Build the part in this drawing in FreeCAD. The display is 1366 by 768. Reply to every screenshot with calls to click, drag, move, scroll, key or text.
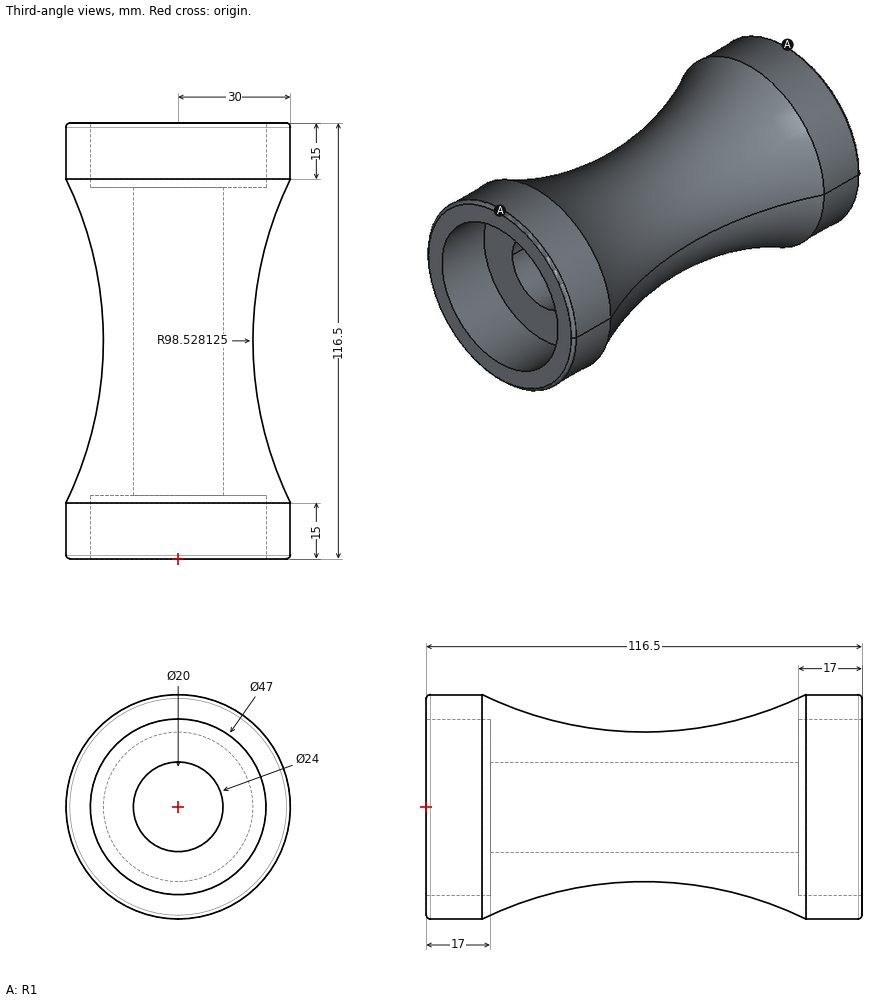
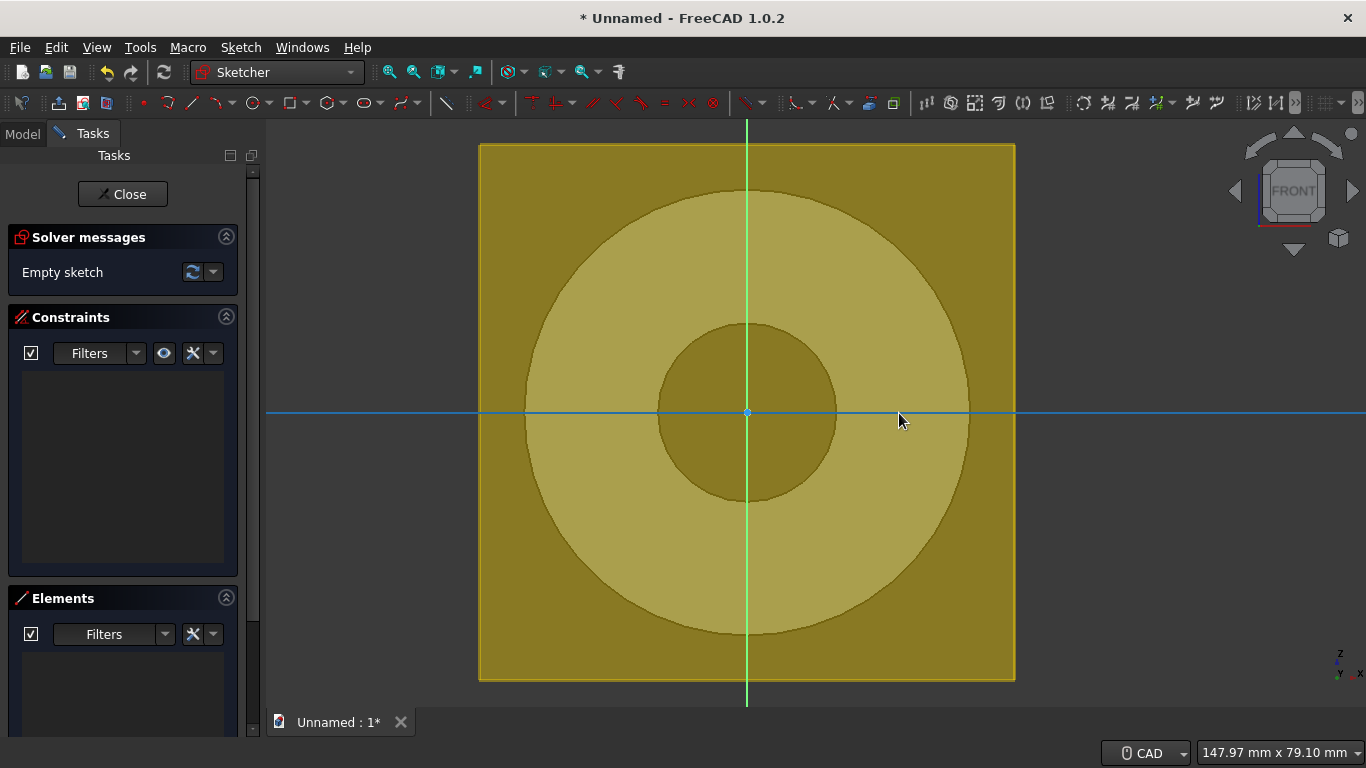
click(254, 104)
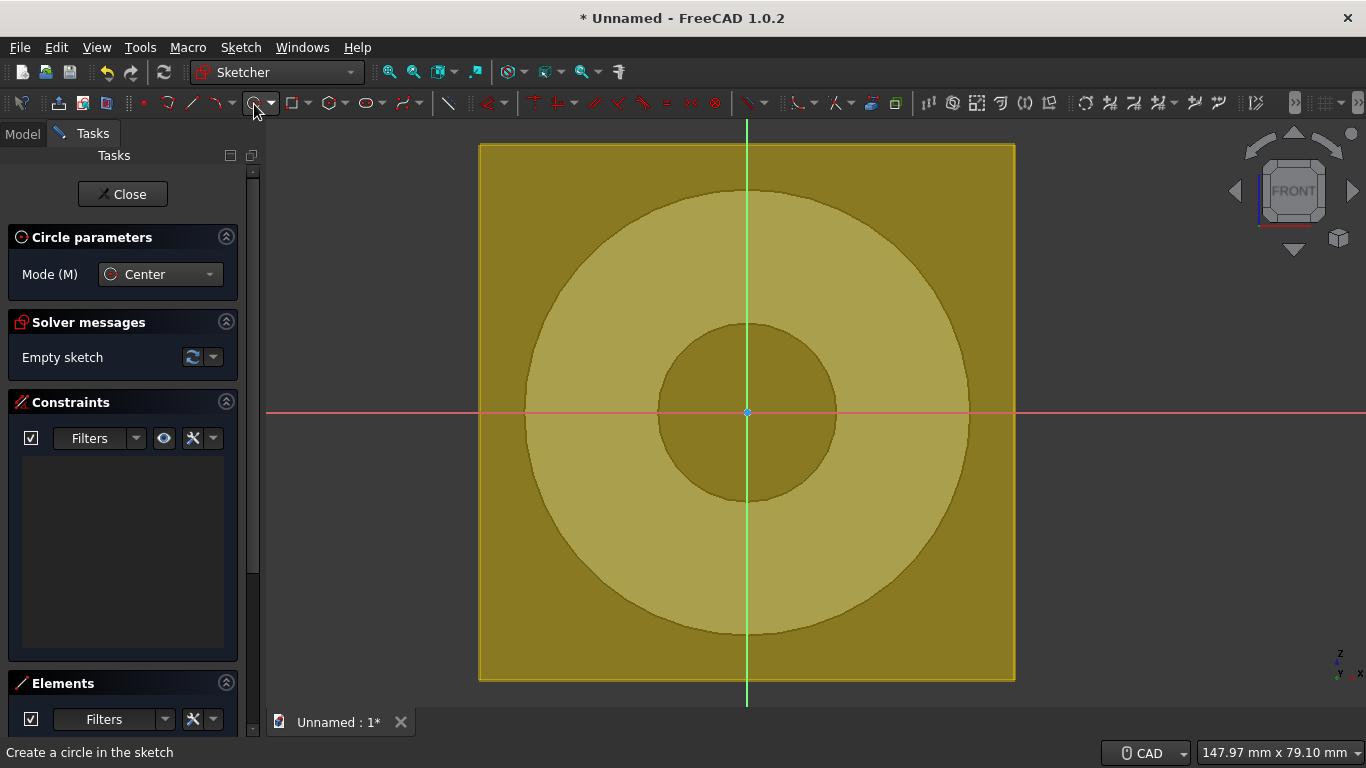
click(747, 413)
click(871, 289)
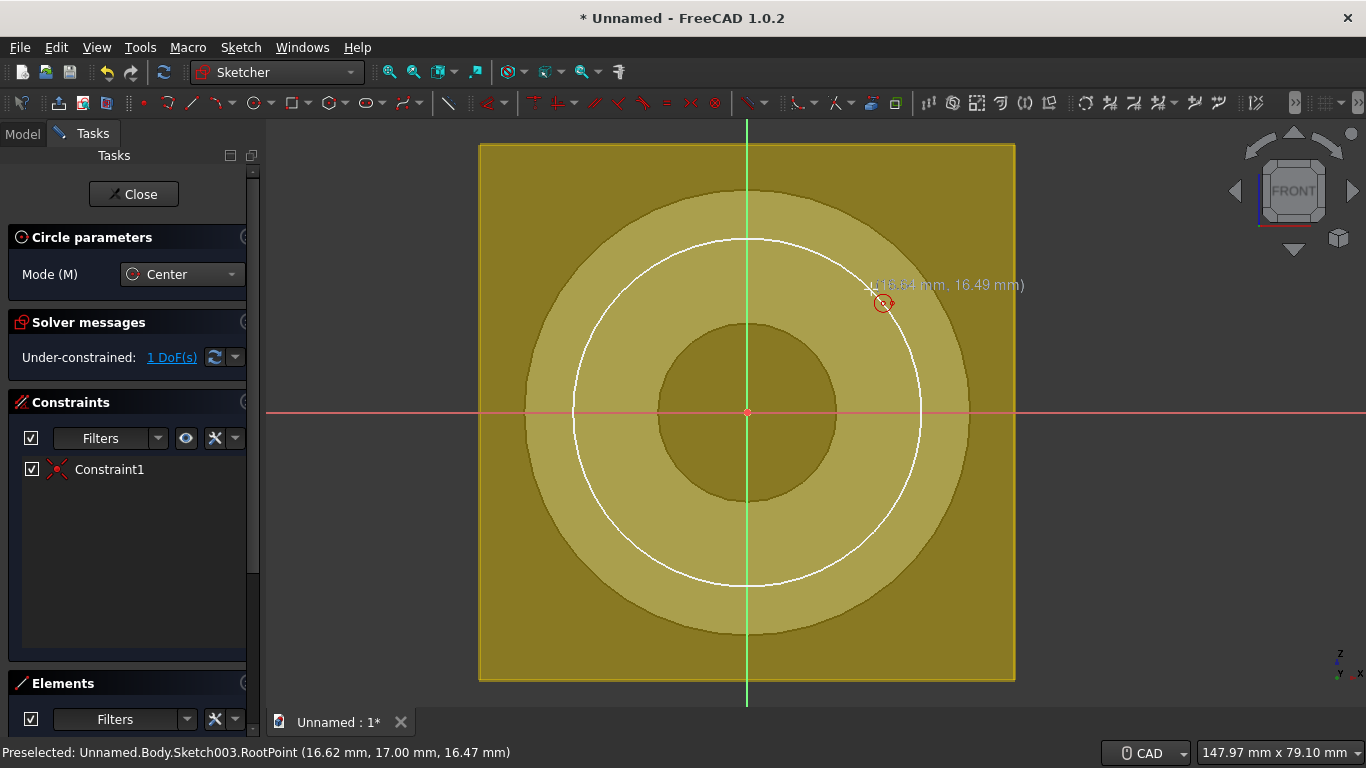
click(747, 413)
click(800, 360)
key(Escape)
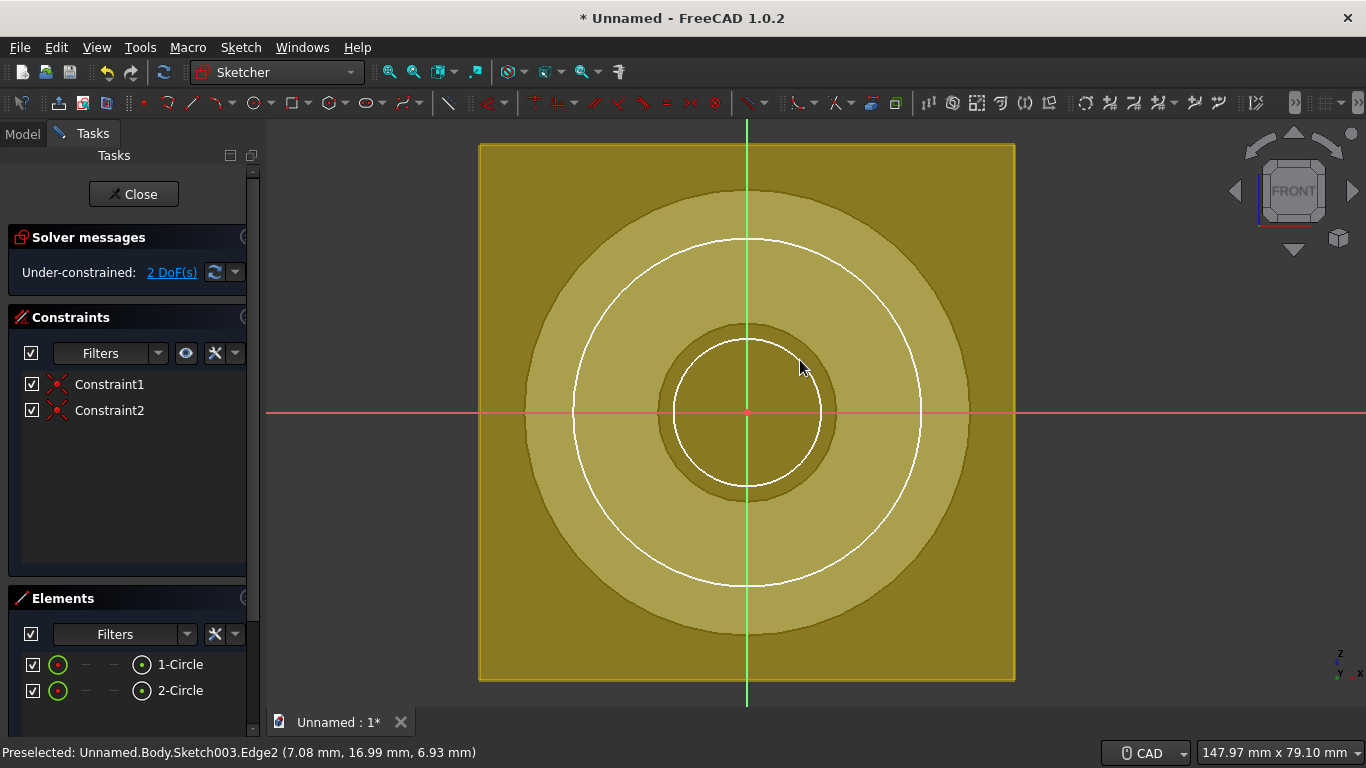
click(488, 104)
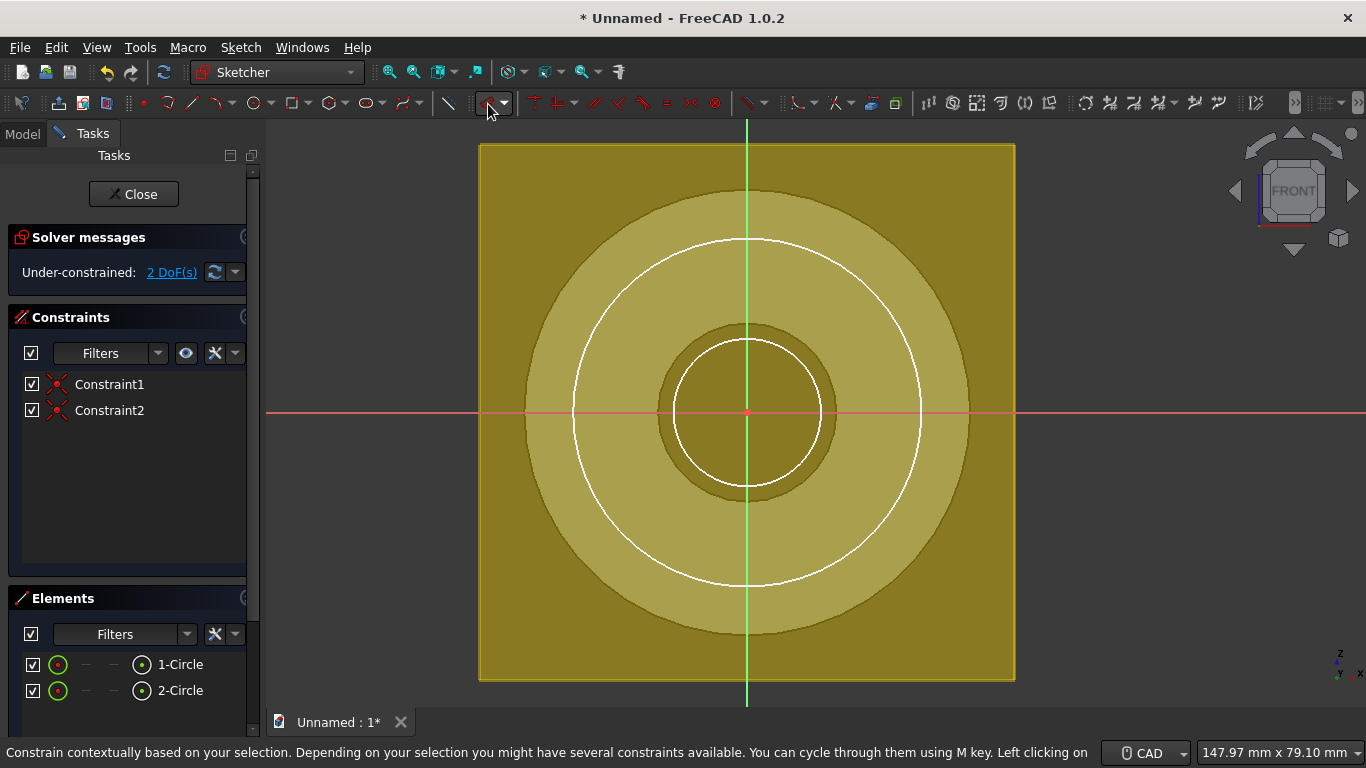
click(870, 289)
click(893, 266)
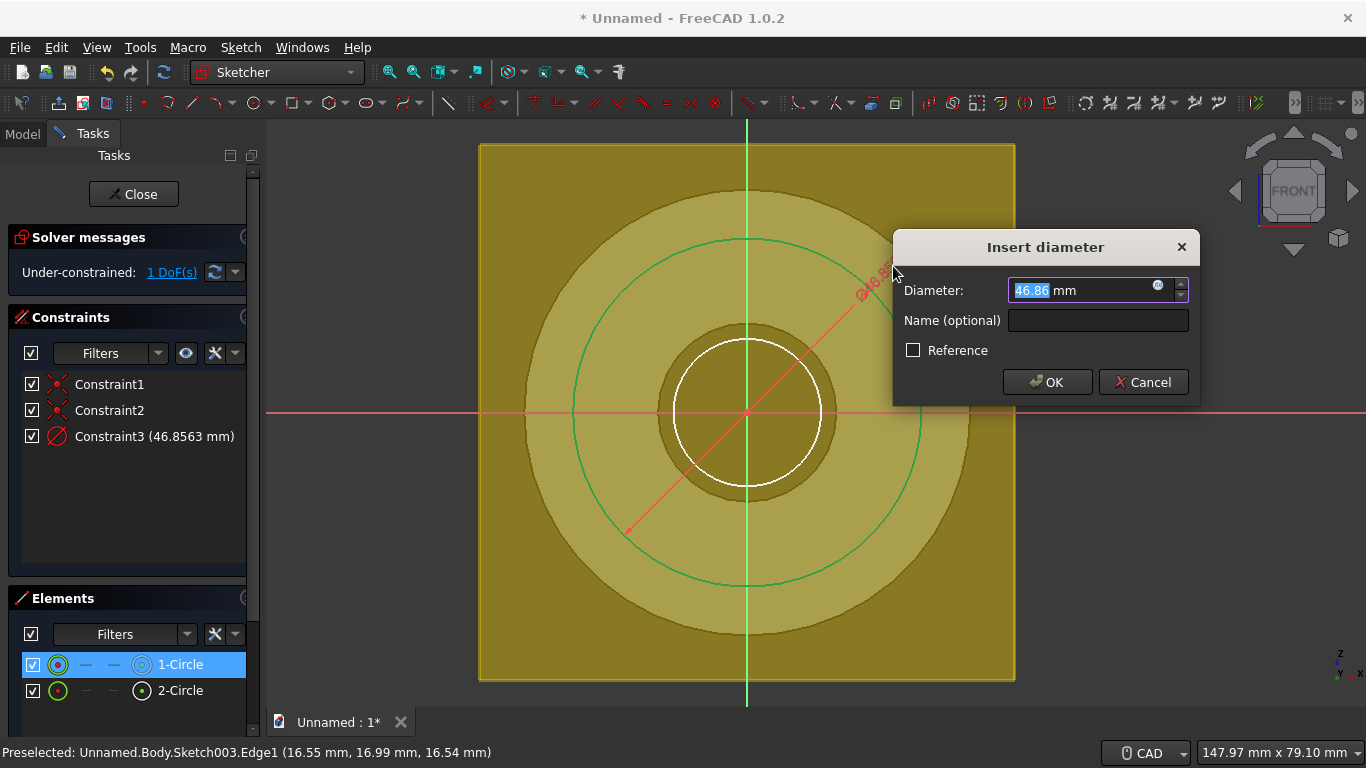
text(47)
key(Return)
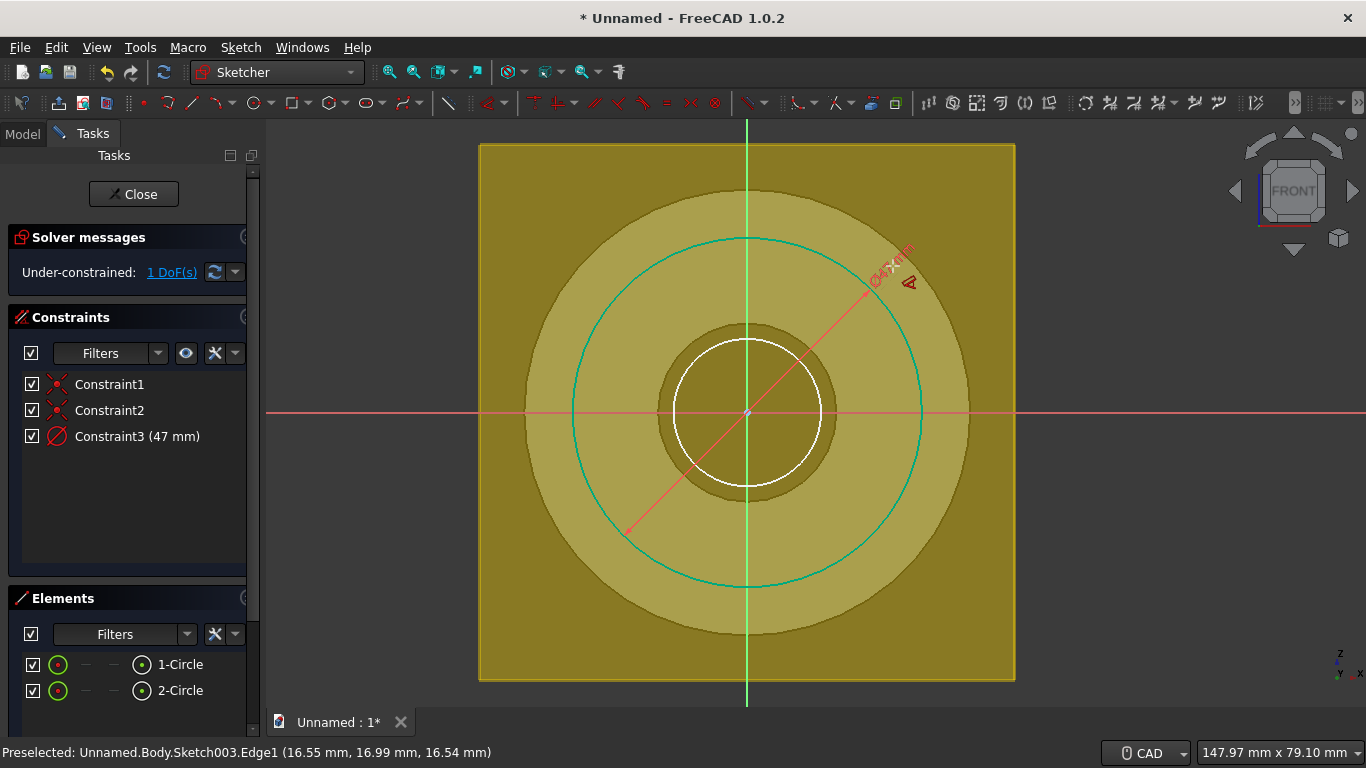
click(799, 360)
click(821, 337)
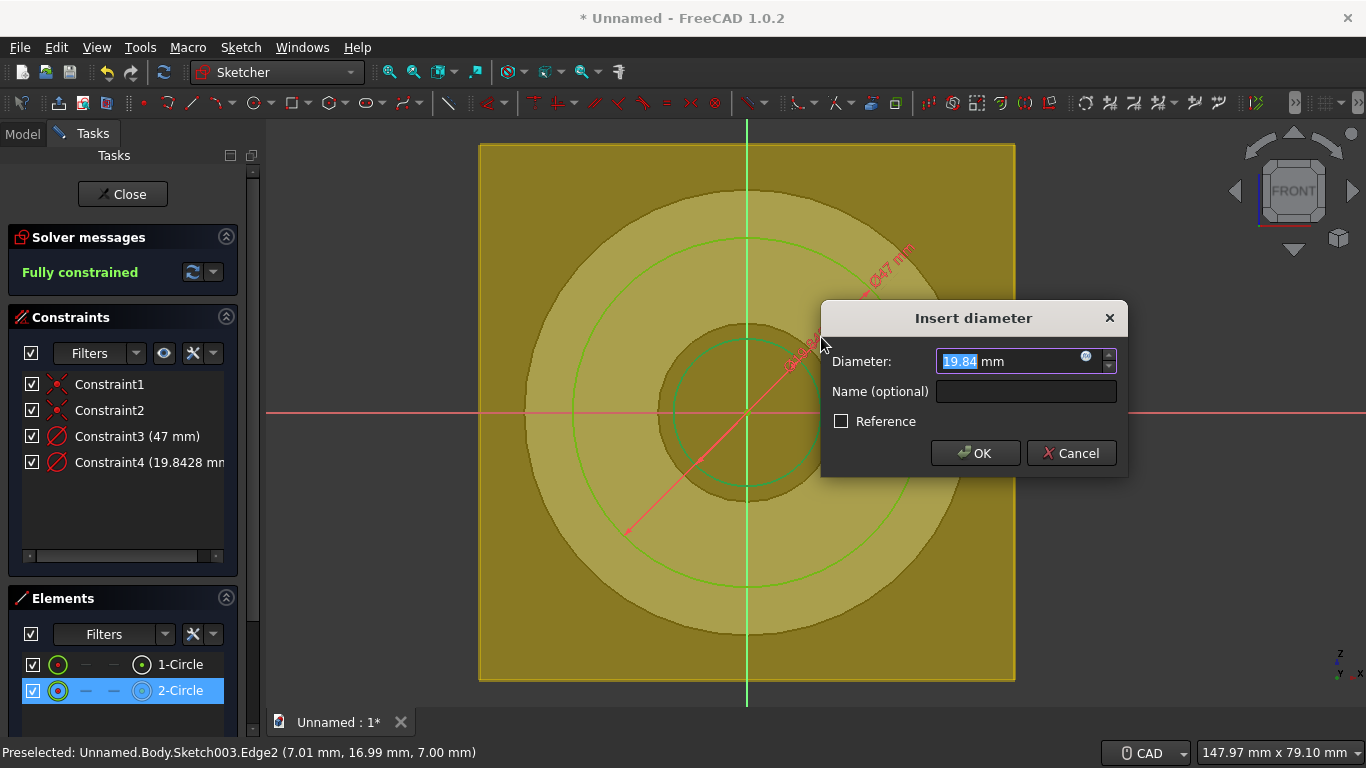
text(20)
key(Return)
key(Escape)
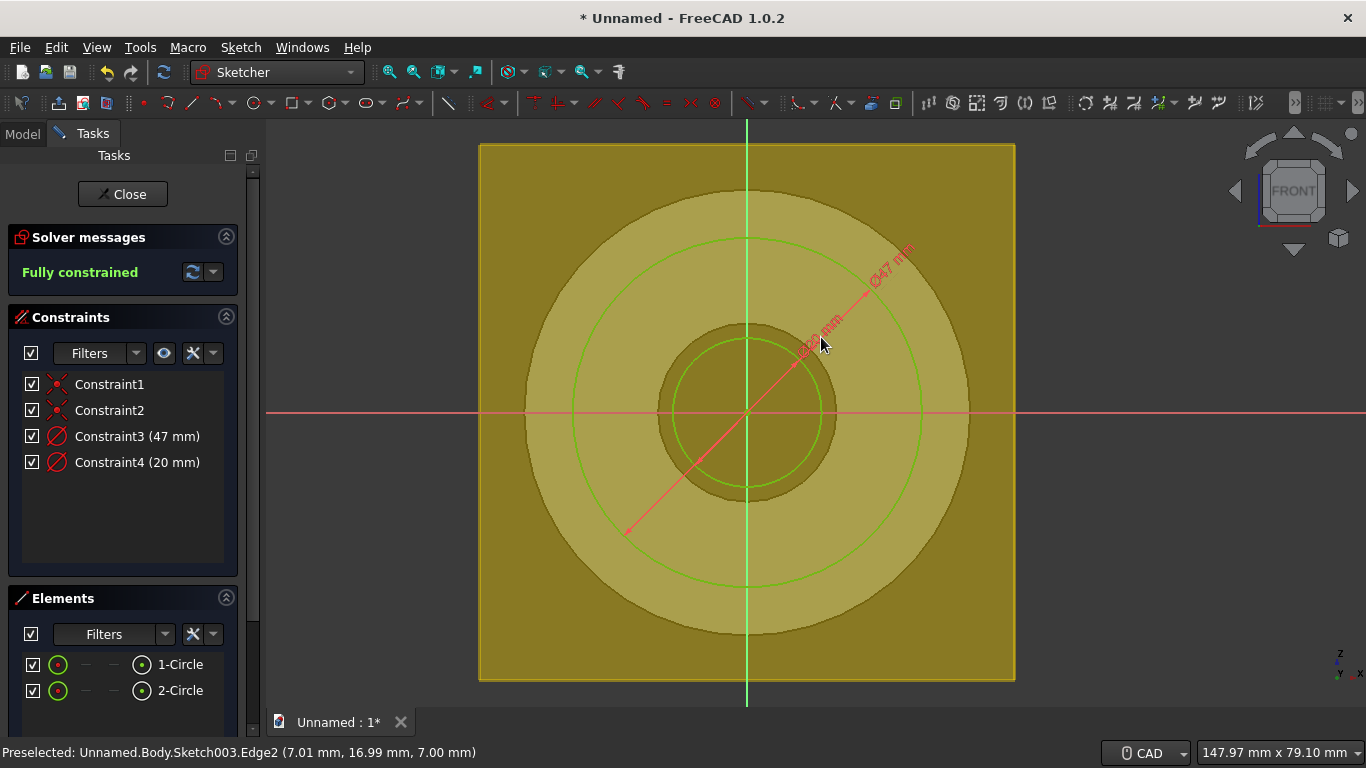
click(123, 194)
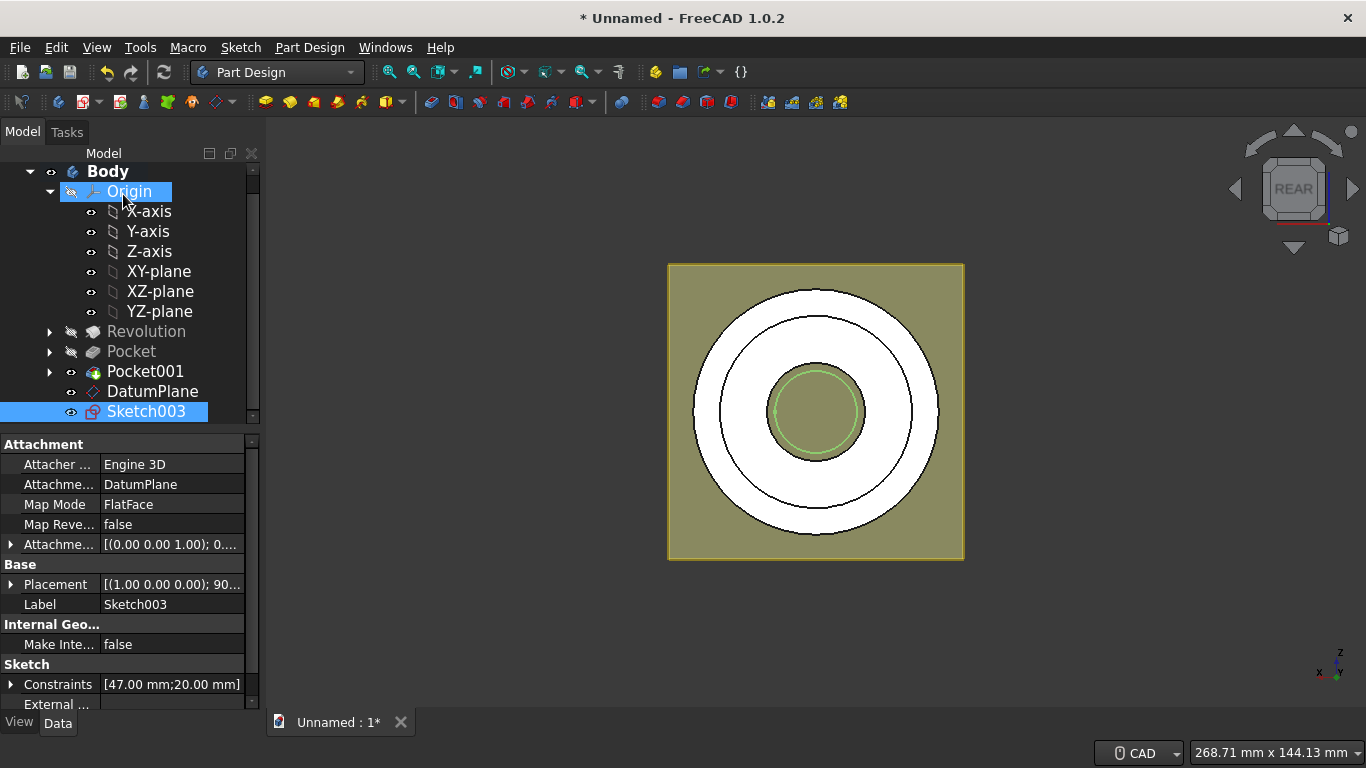
click(432, 102)